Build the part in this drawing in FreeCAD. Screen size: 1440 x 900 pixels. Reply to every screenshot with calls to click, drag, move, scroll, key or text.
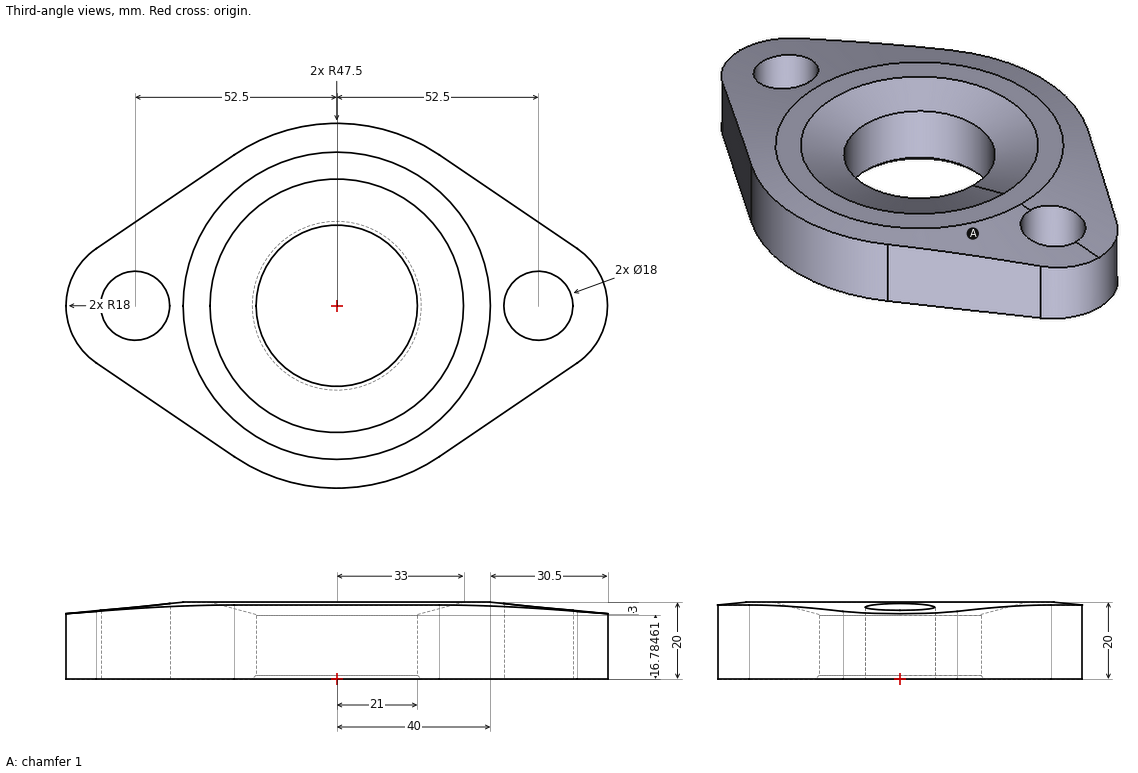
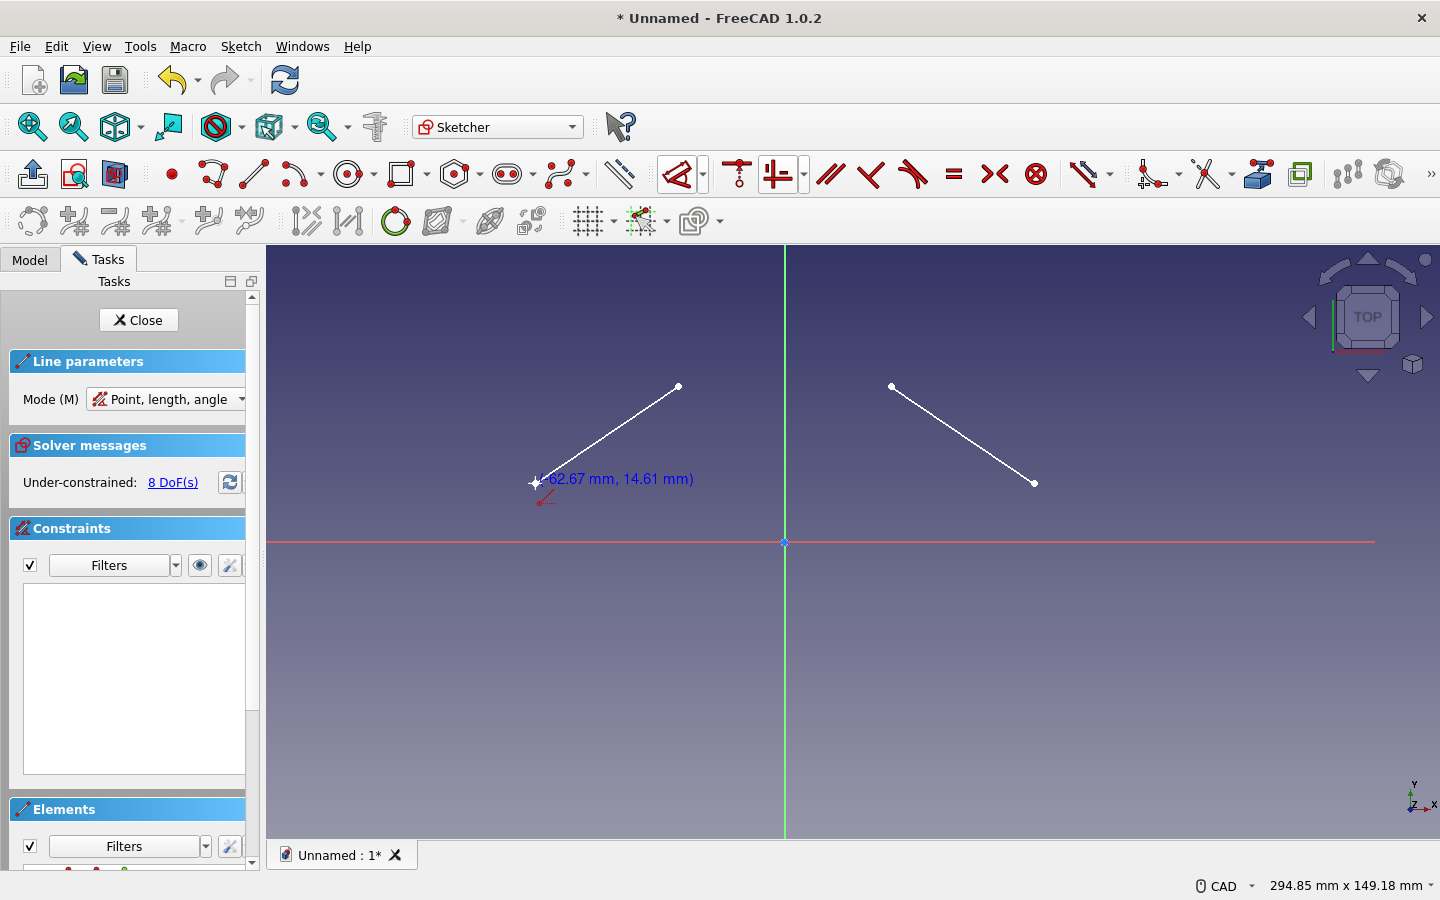
click(535, 601)
click(678, 699)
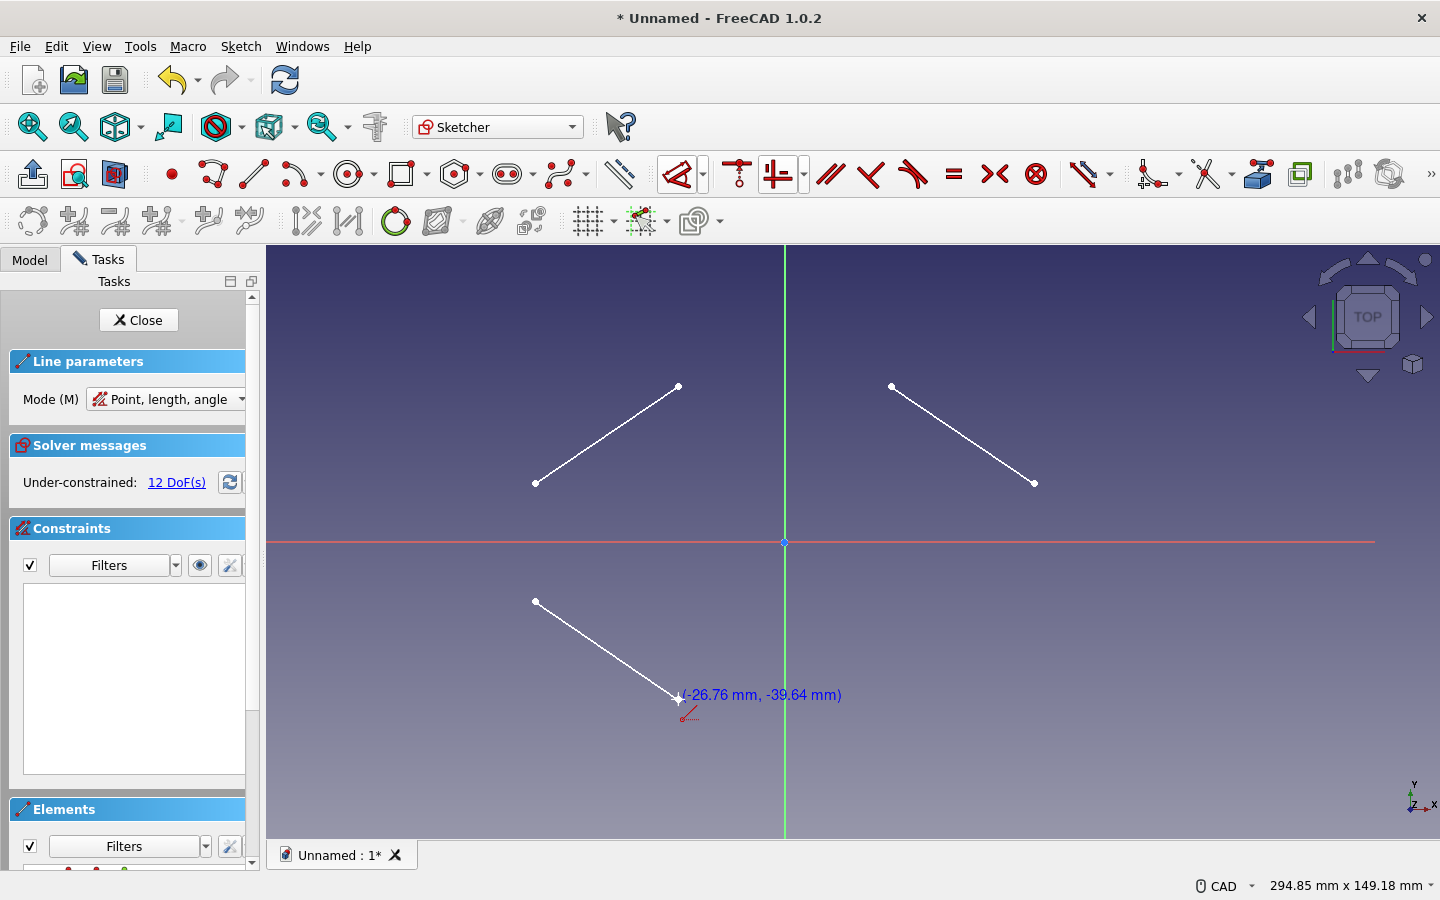
click(891, 699)
click(1034, 601)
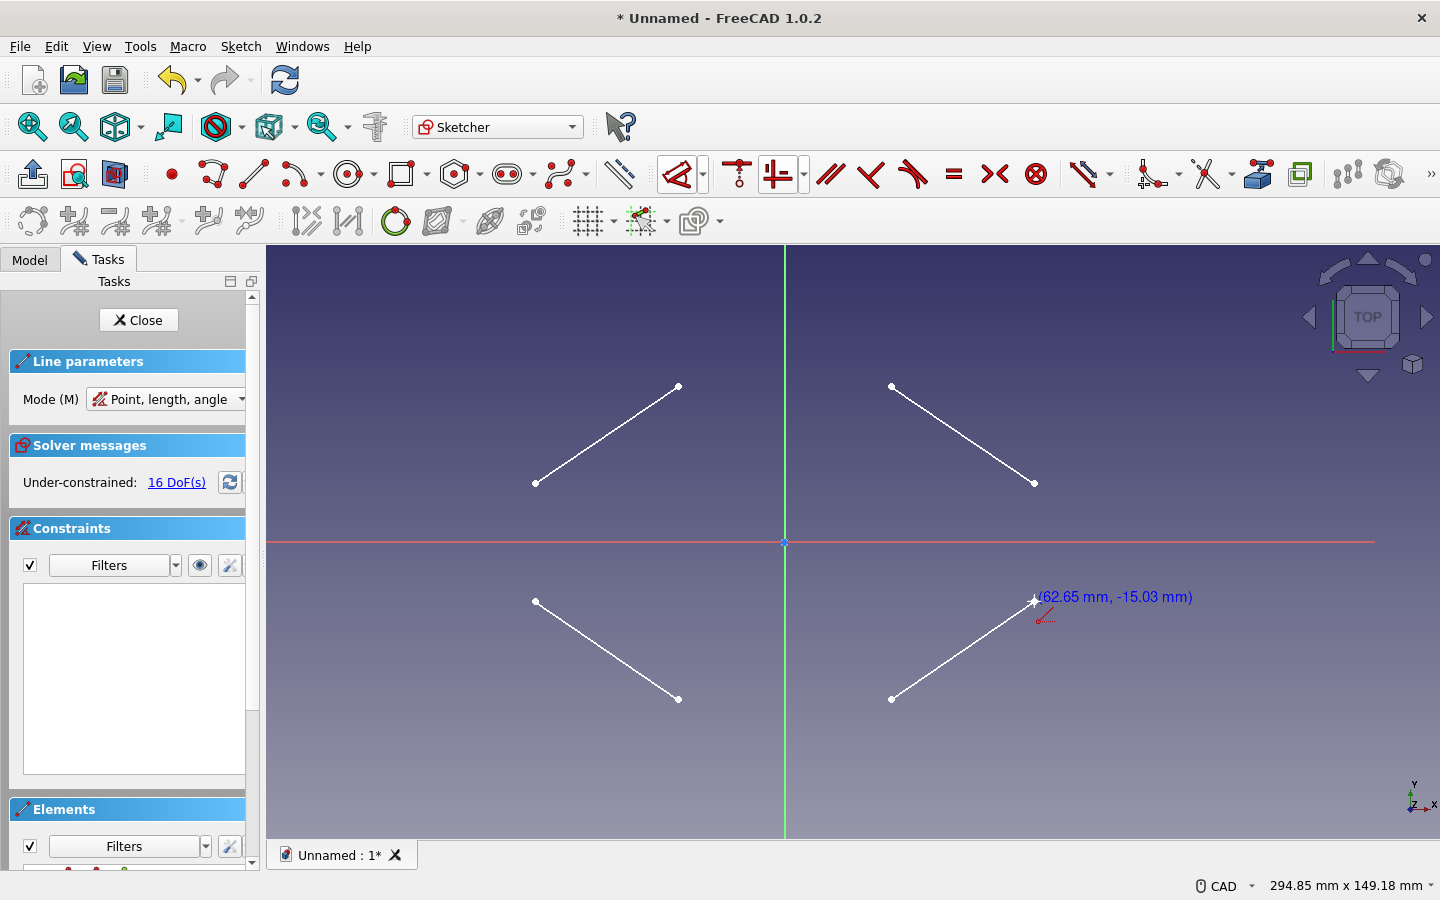
key(g)
key(3)
key(a)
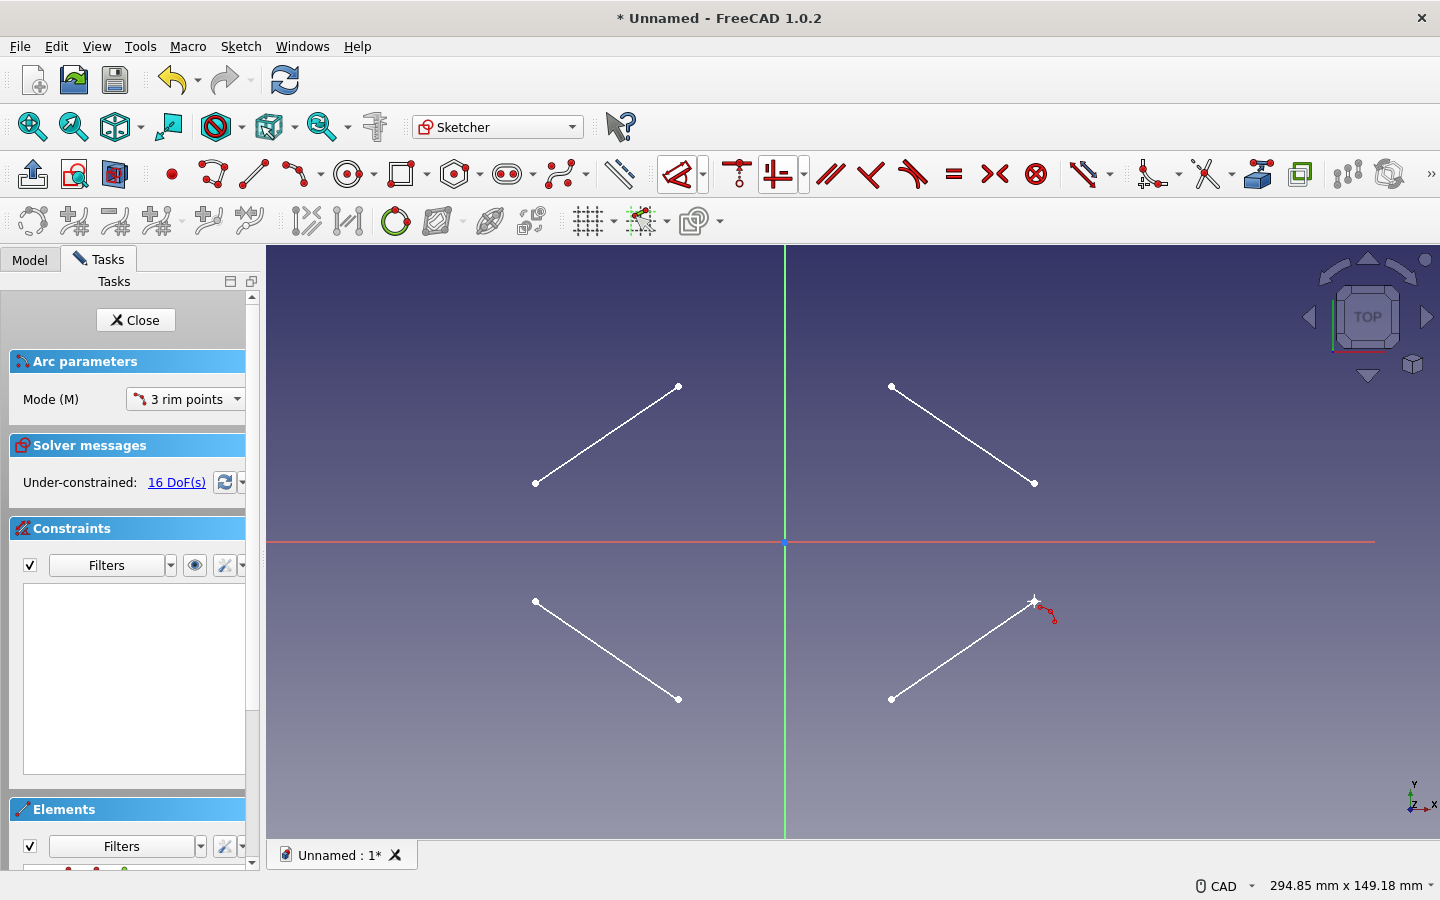
click(891, 387)
click(678, 387)
click(807, 354)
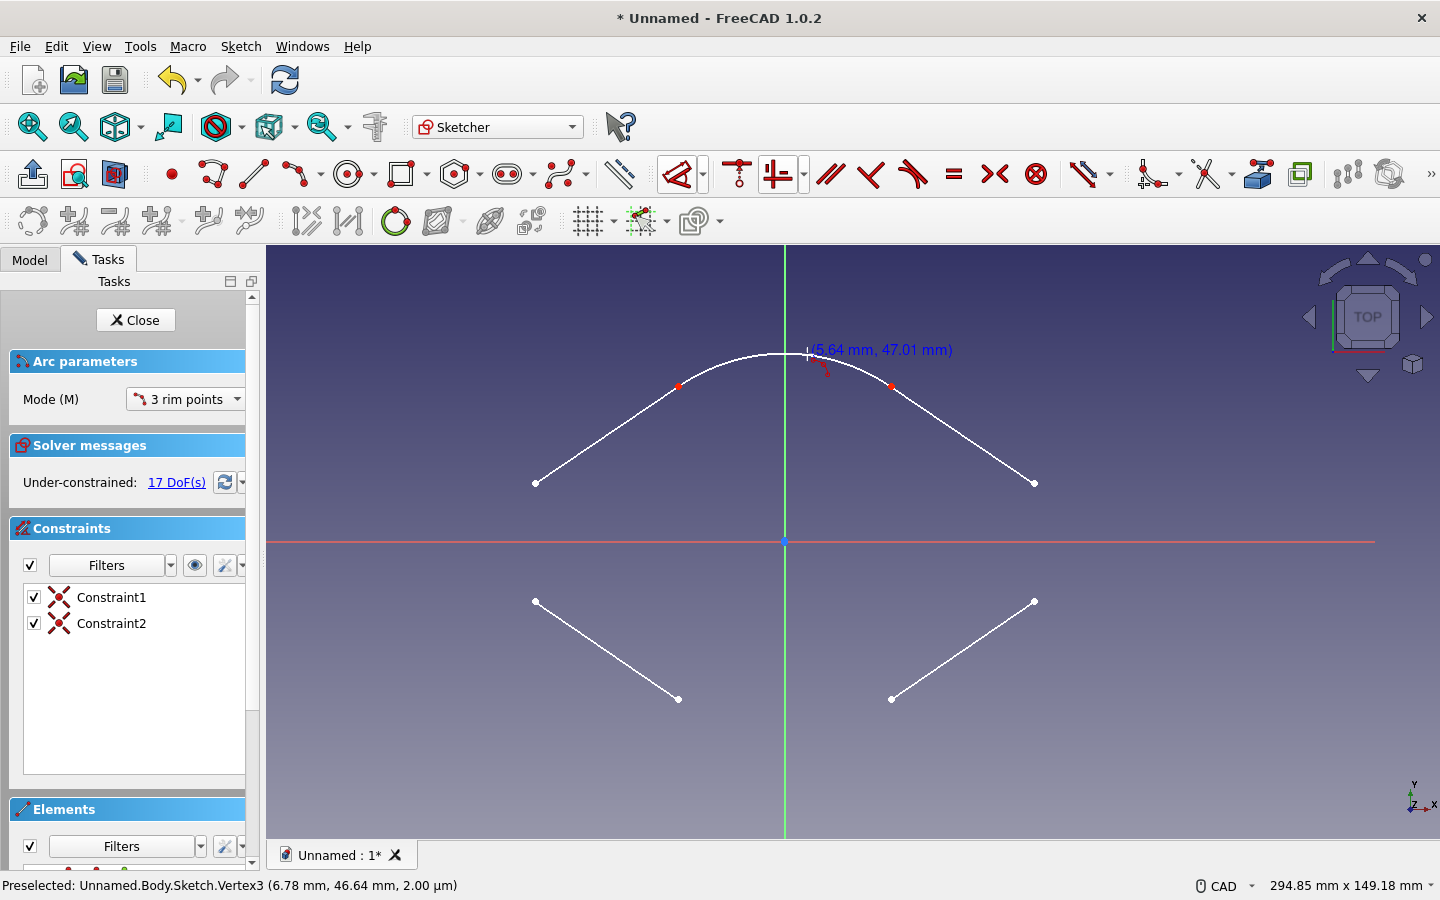
click(535, 484)
click(535, 602)
click(509, 515)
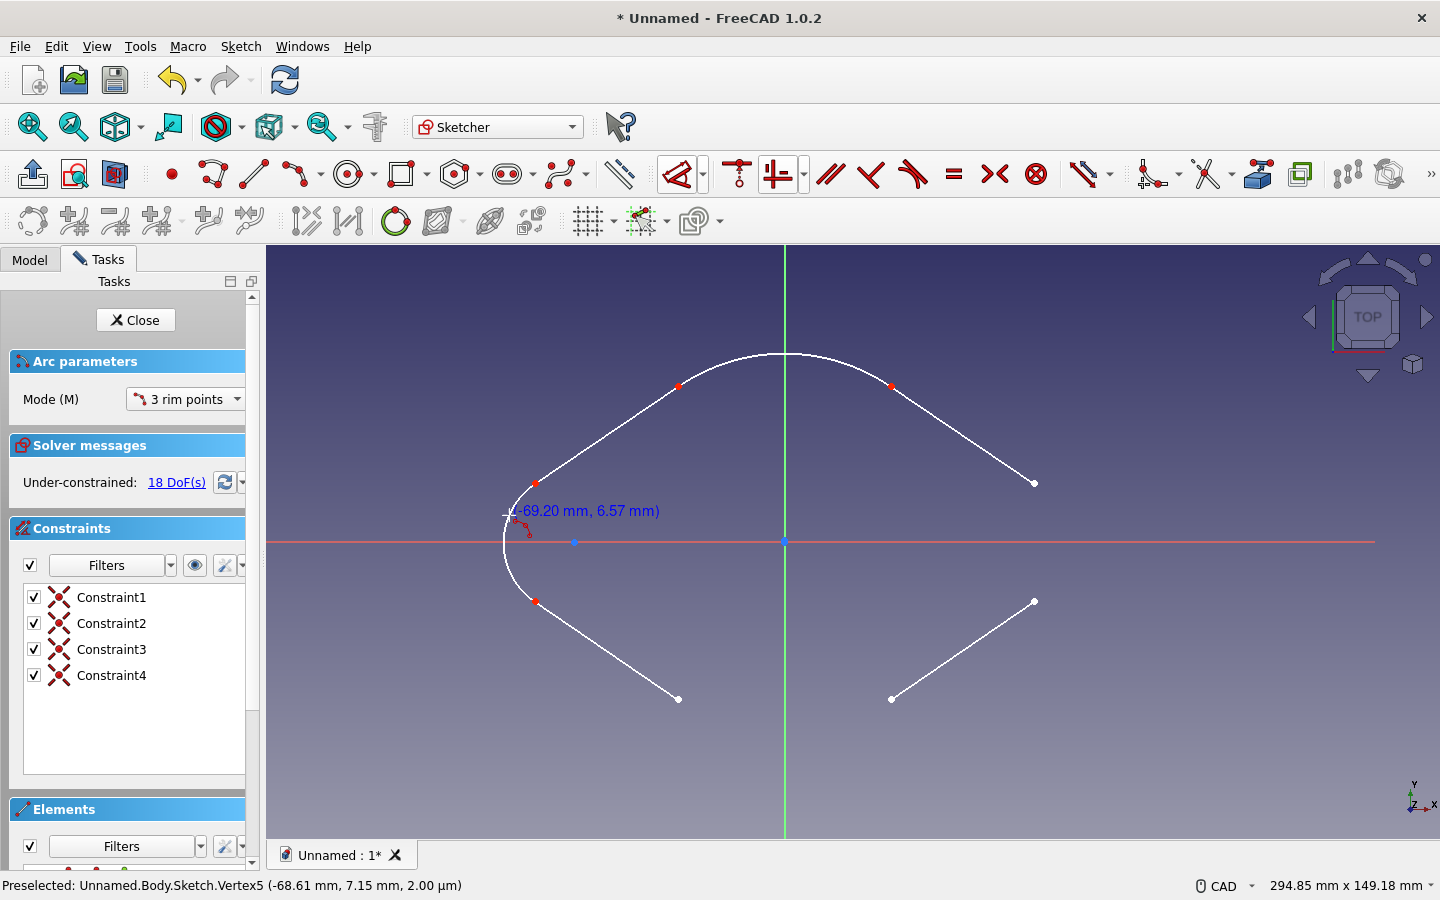
click(678, 700)
click(891, 700)
click(762, 730)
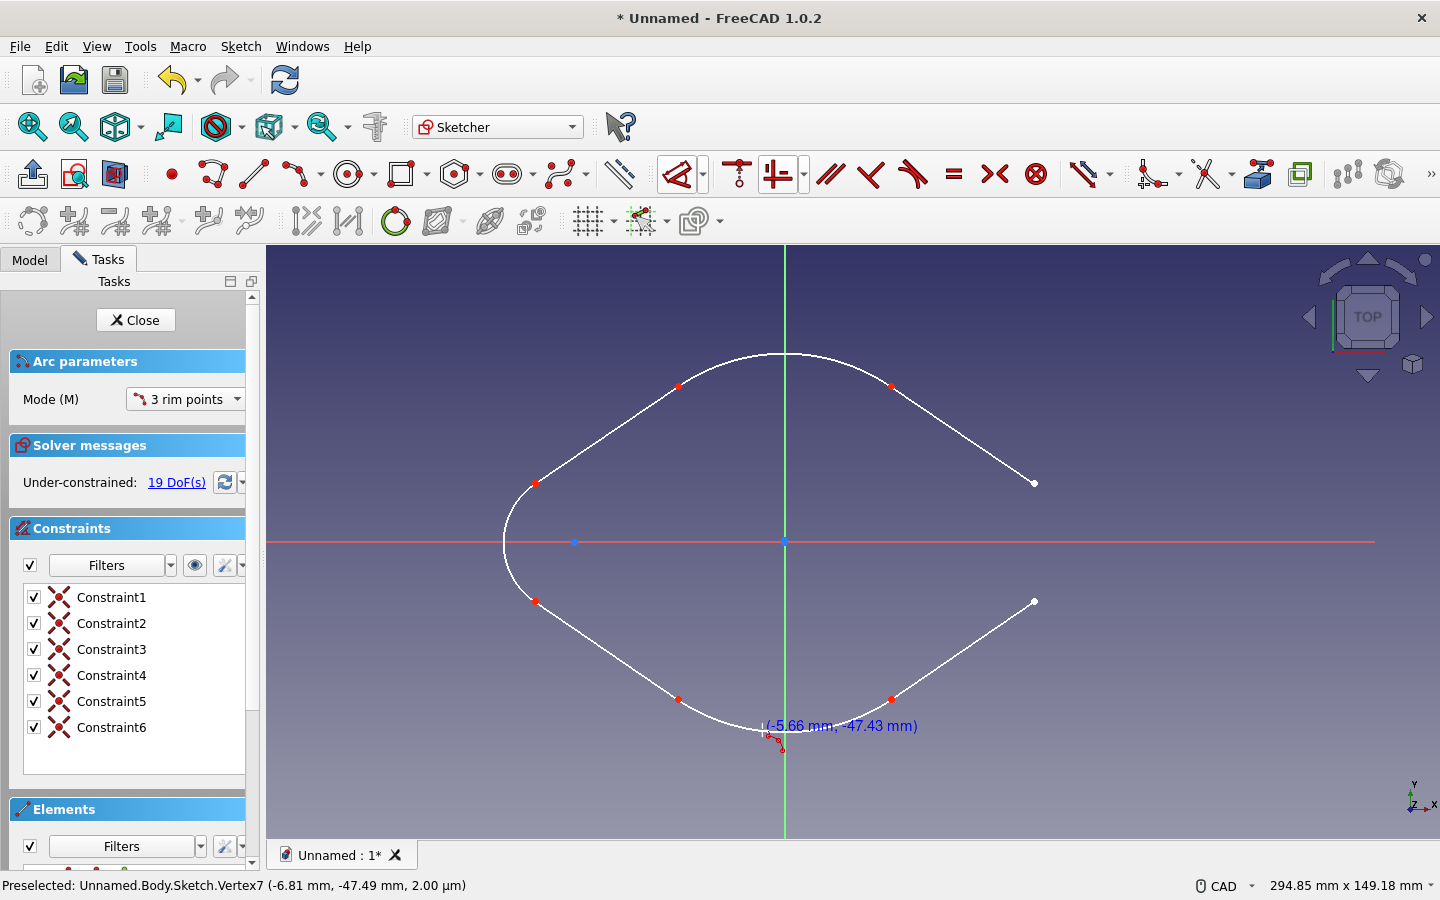
click(1034, 602)
click(1034, 484)
click(1060, 569)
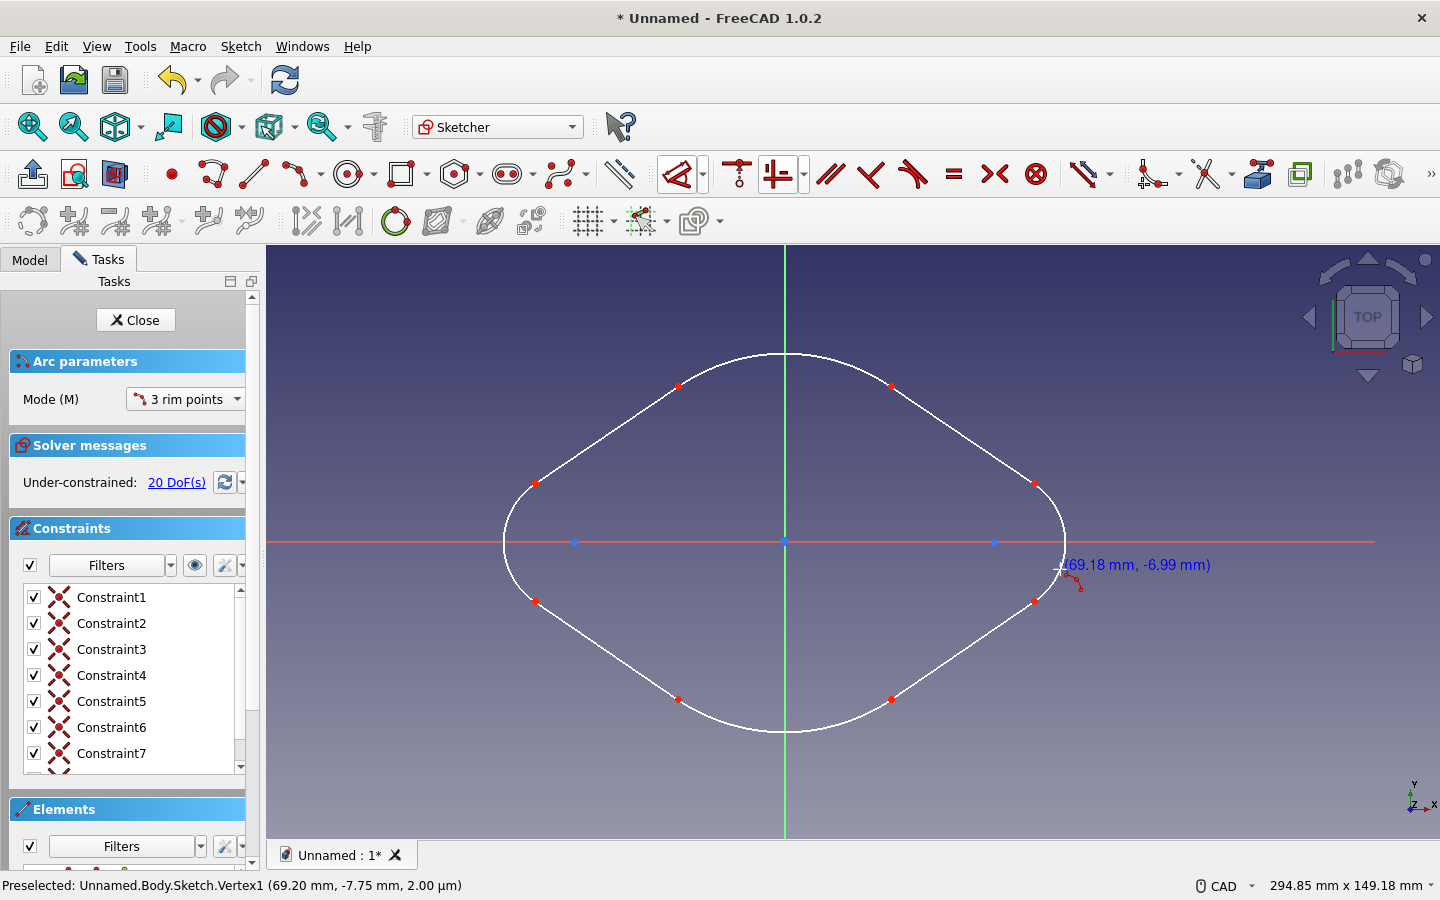
click(348, 174)